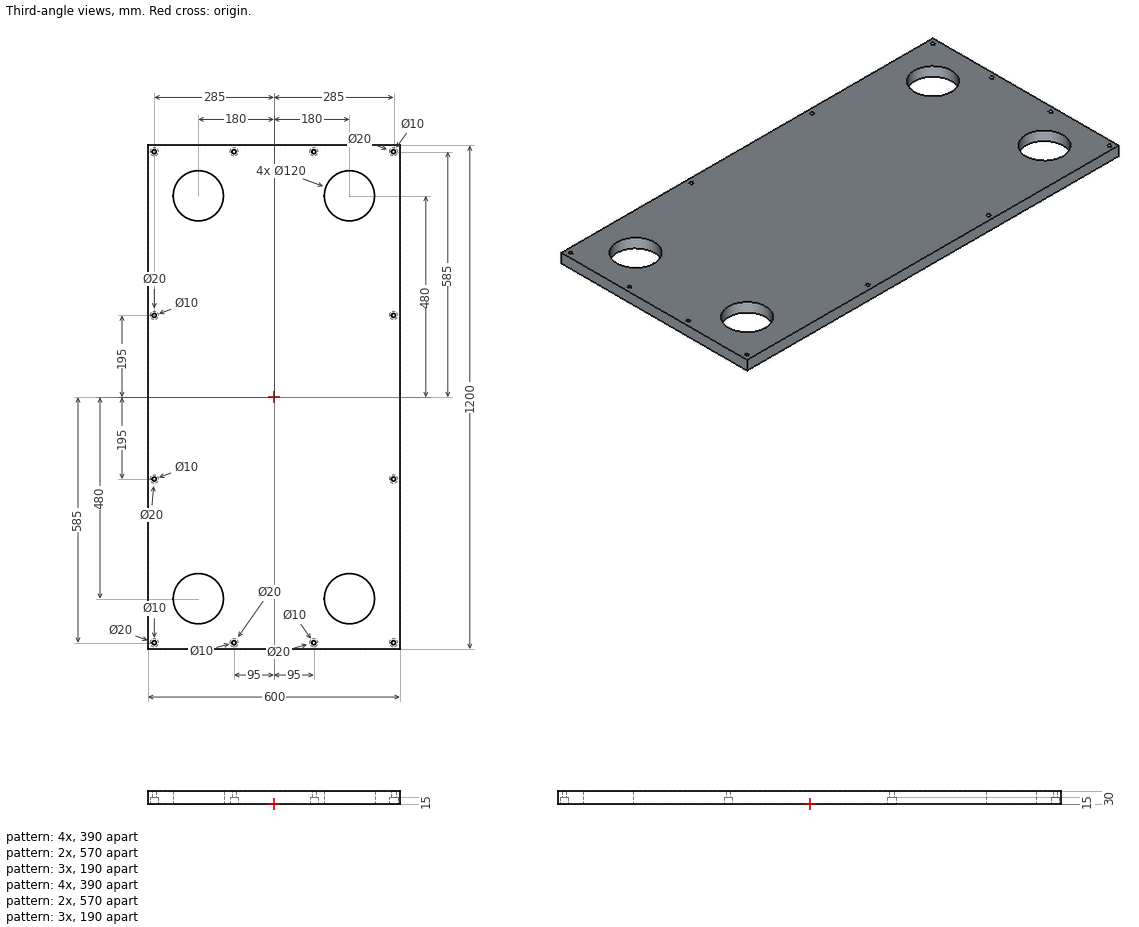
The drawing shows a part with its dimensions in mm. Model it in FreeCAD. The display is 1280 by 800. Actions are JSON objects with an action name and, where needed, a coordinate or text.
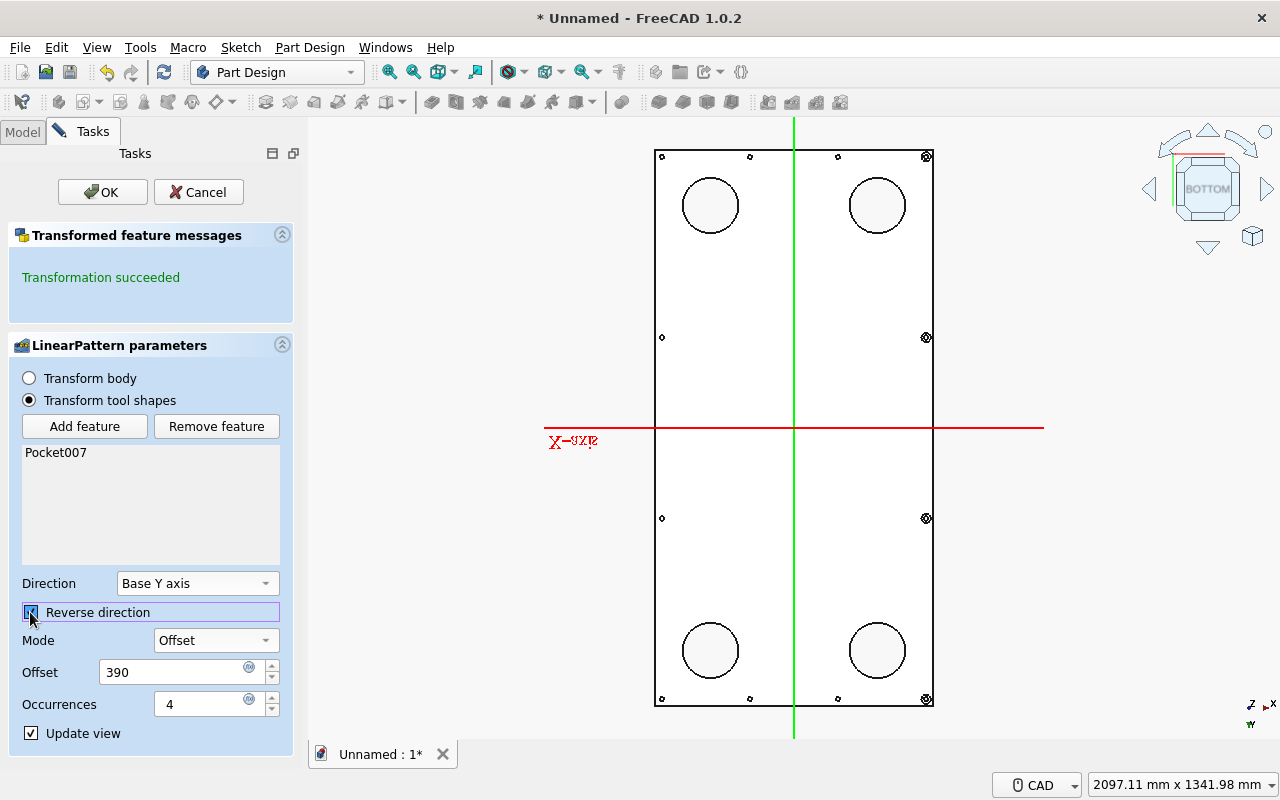
{"action": "left_click", "coordinate": [103, 192]}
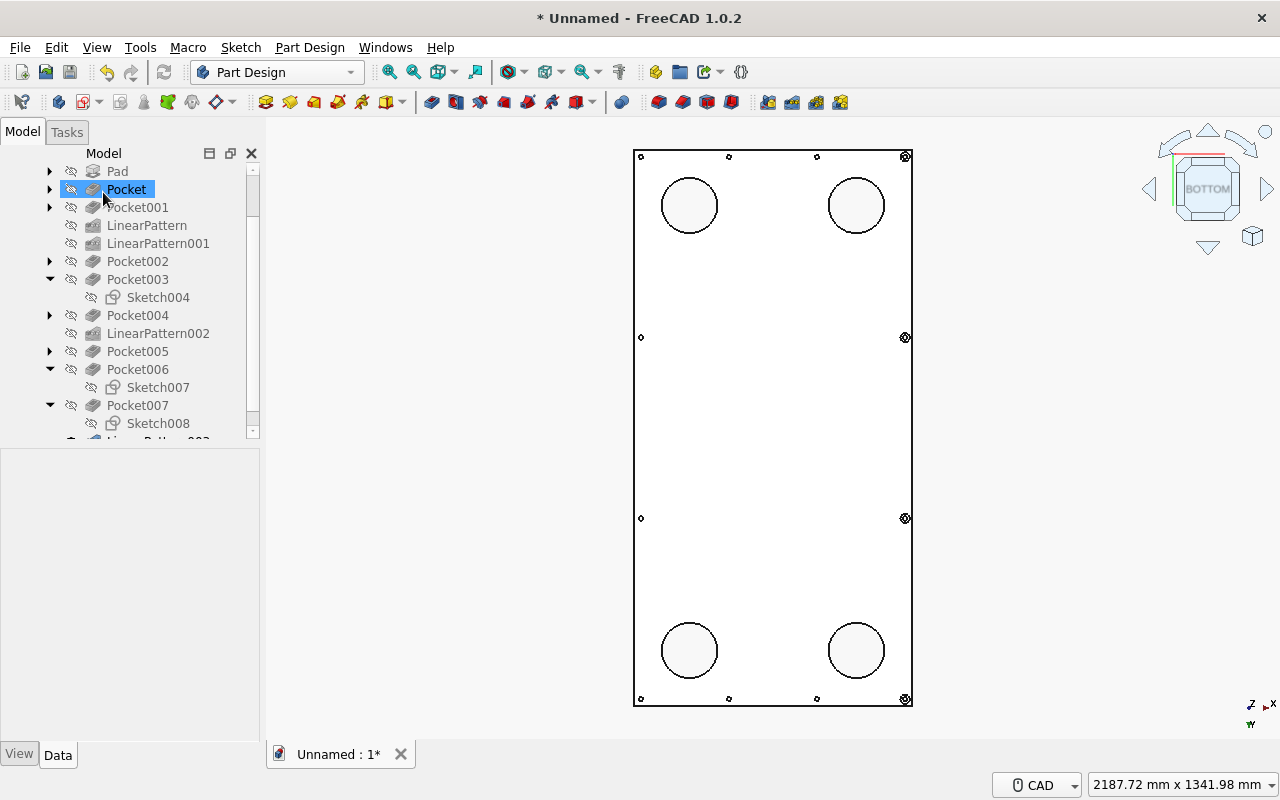
{"action": "left_click", "coordinate": [116, 405]}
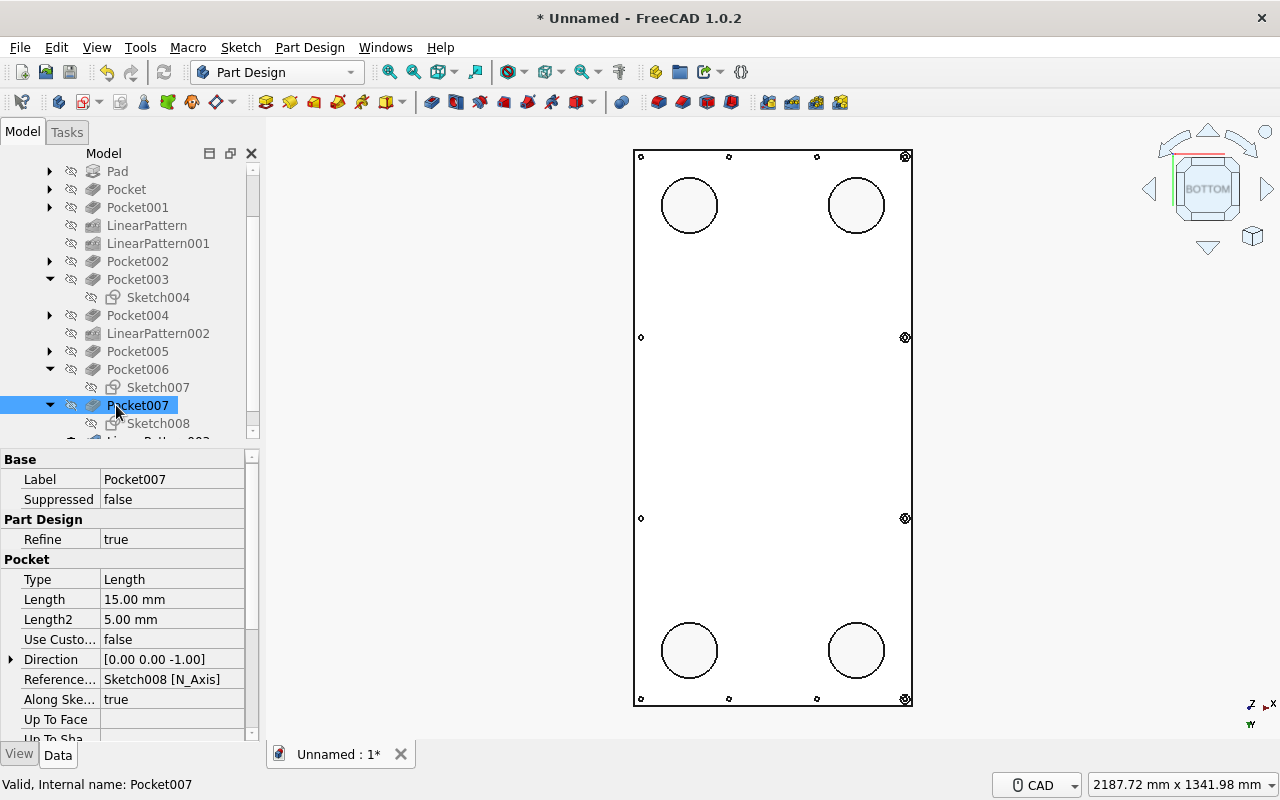
{"action": "left_click", "coordinate": [792, 102]}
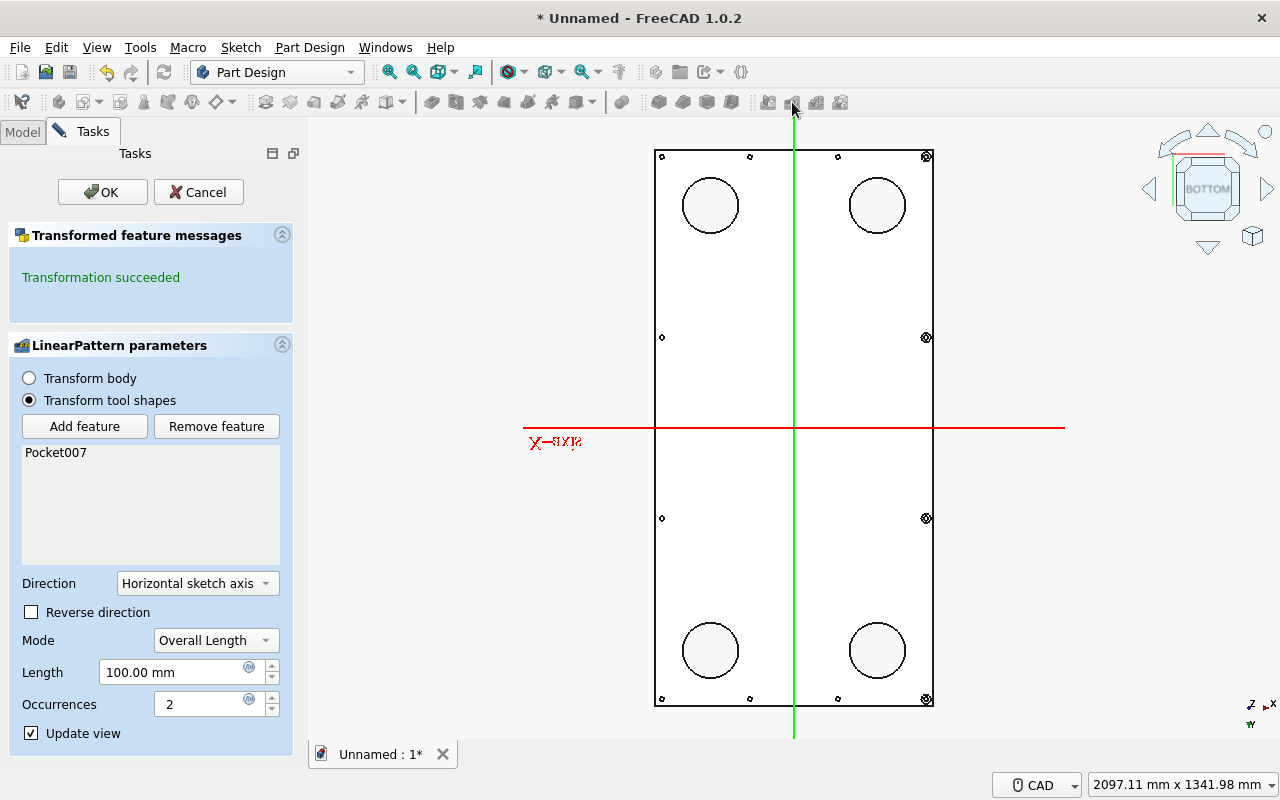
{"action": "left_click", "coordinate": [198, 584]}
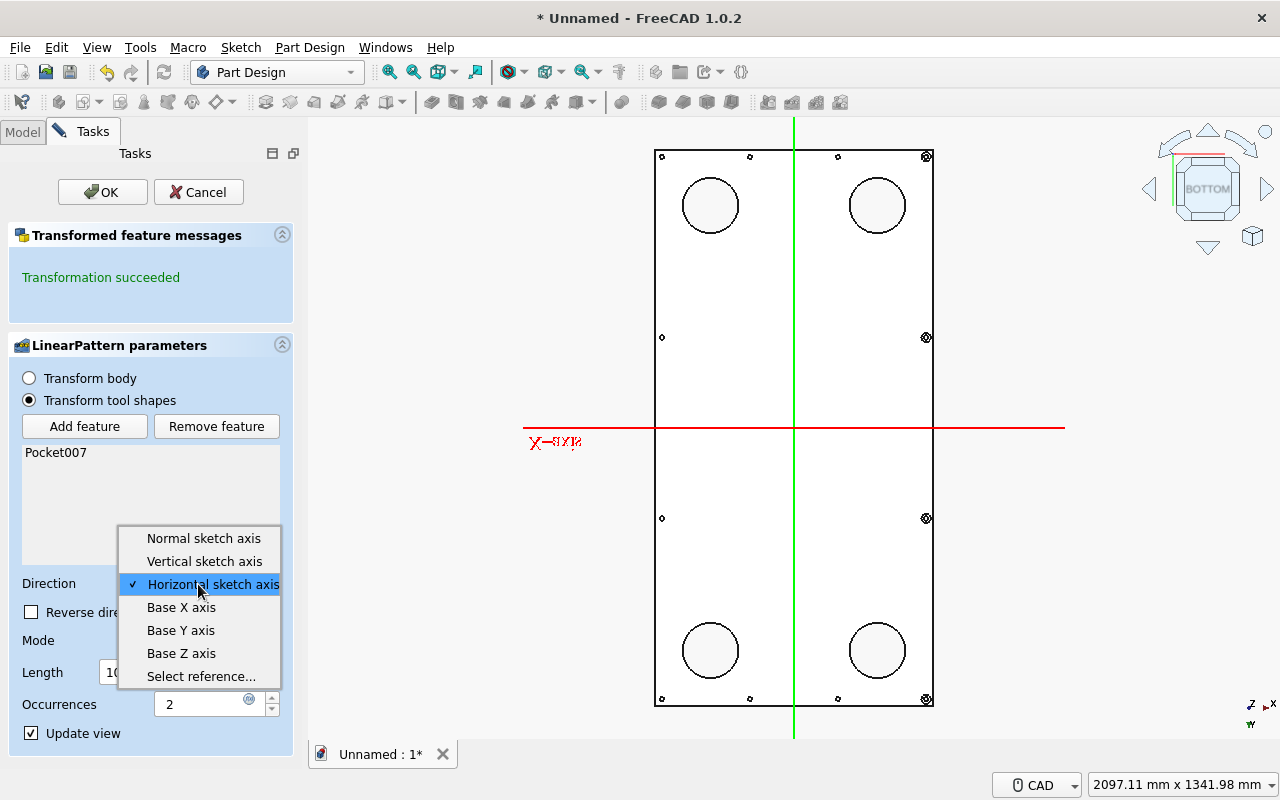
{"action": "left_click", "coordinate": [198, 608]}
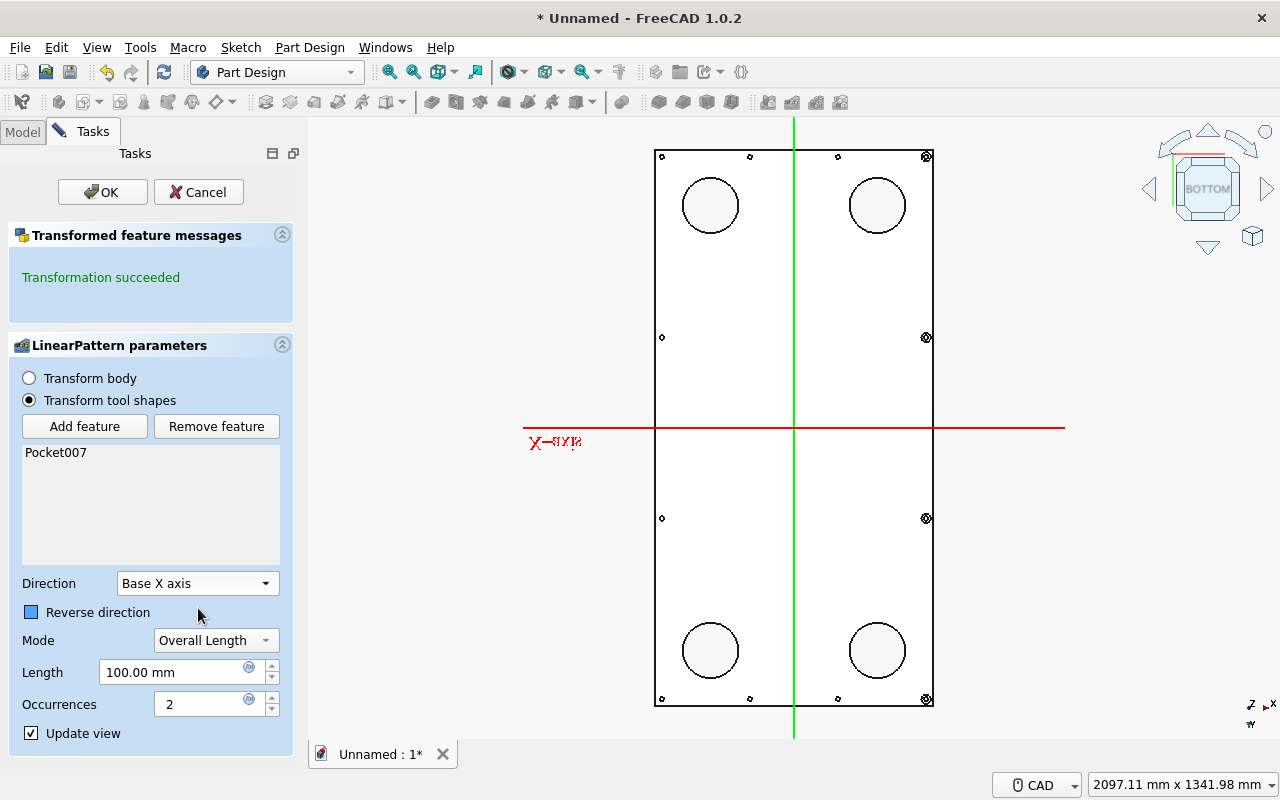
{"action": "left_click", "coordinate": [217, 640]}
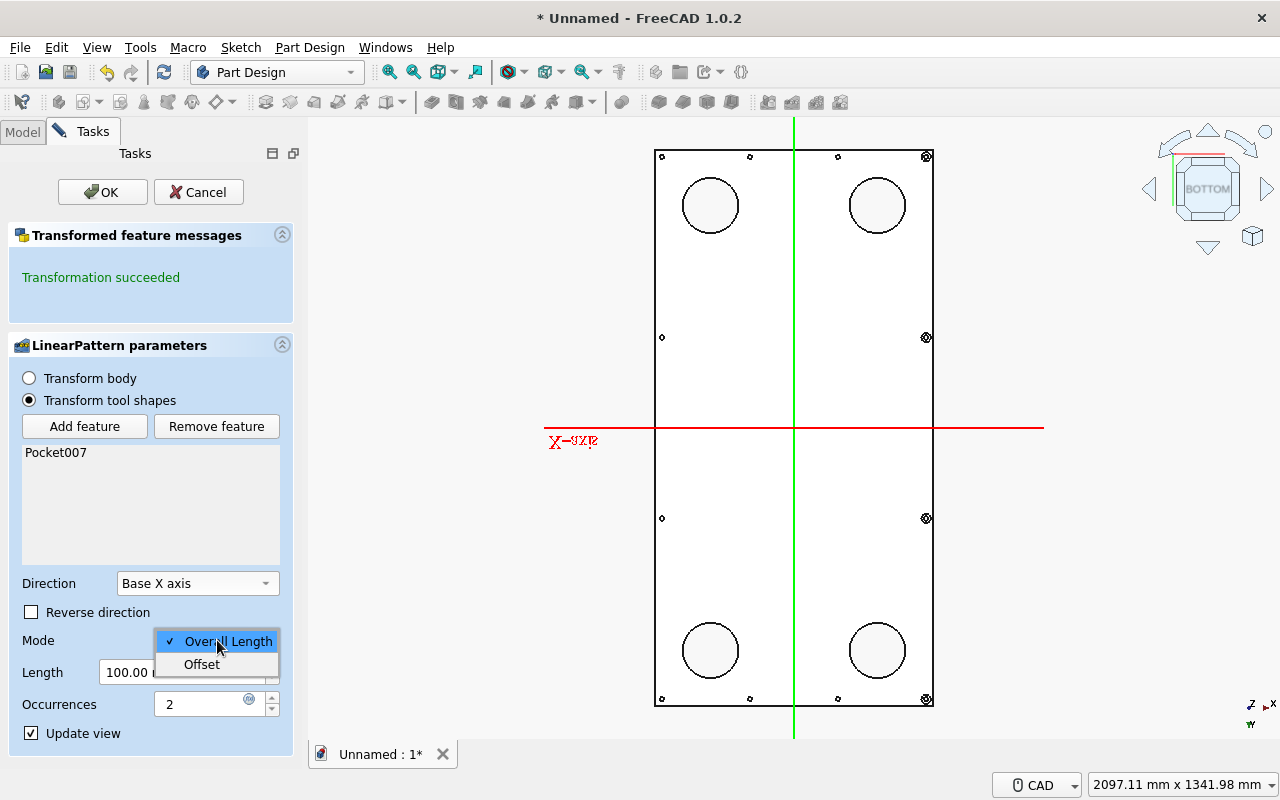
{"action": "left_click", "coordinate": [216, 664]}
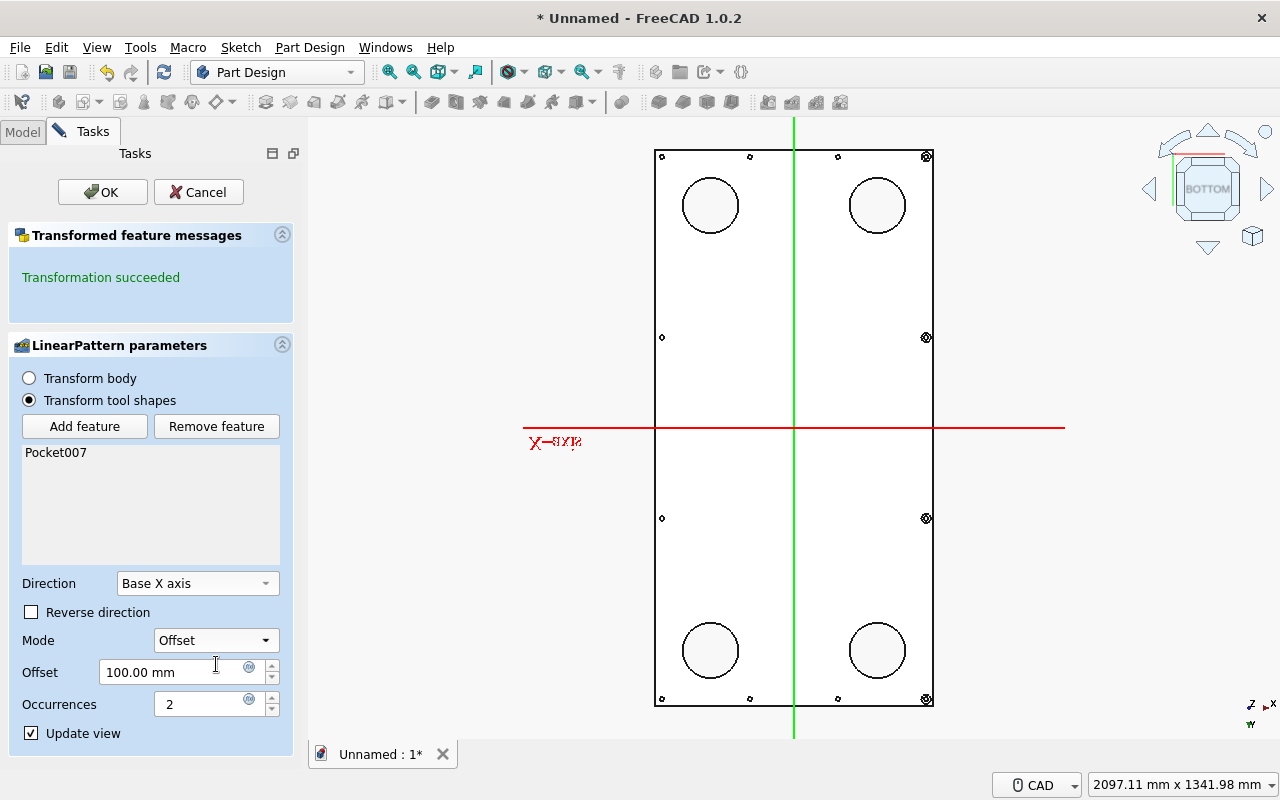
{"action": "triple_click", "coordinate": [182, 672]}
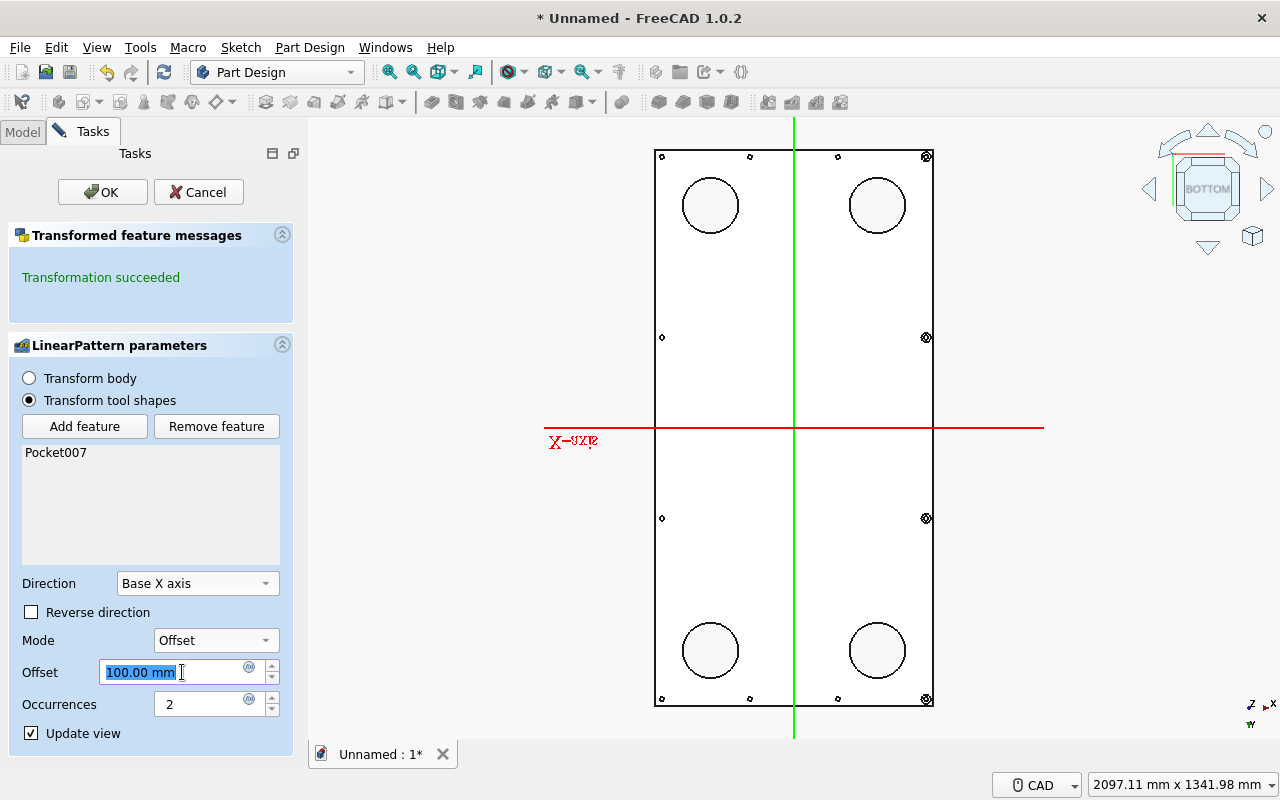
{"action": "type", "text": "570"}
{"action": "key", "text": "Tab"}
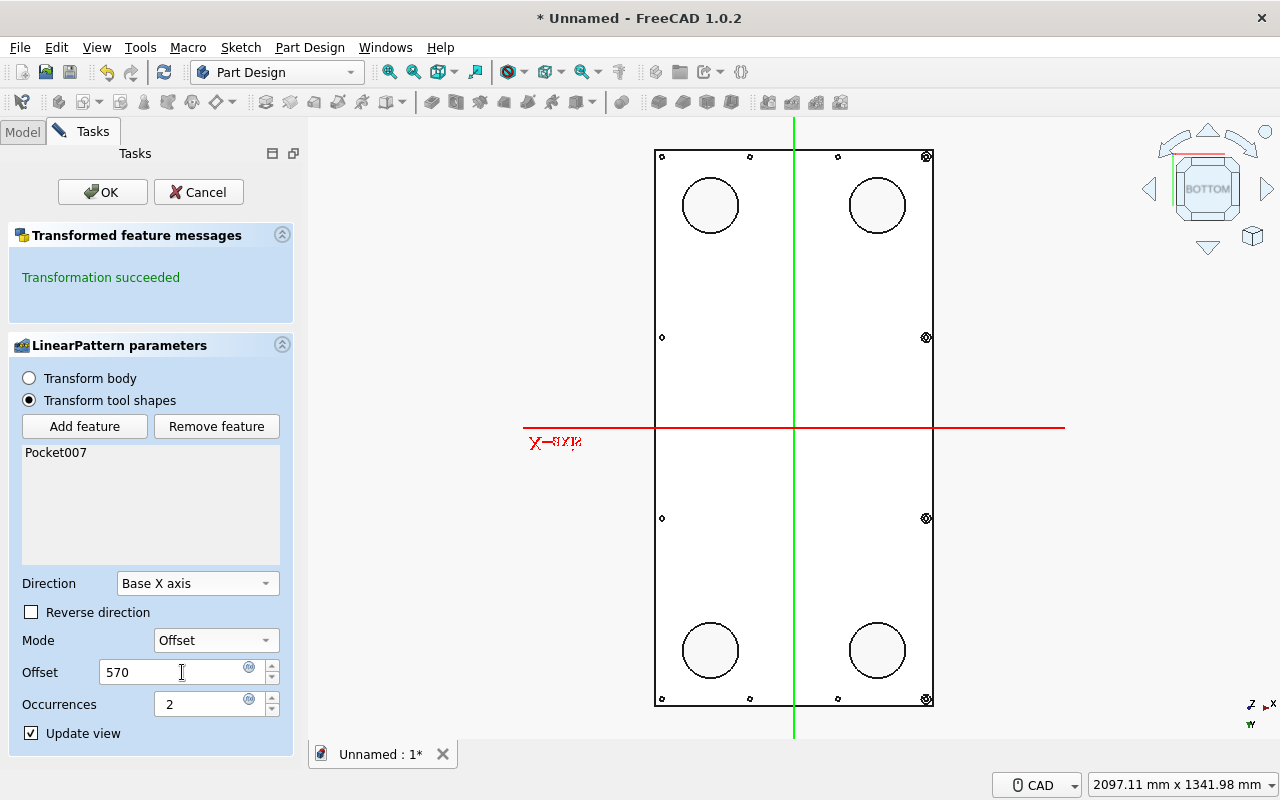
{"action": "triple_click", "coordinate": [209, 704]}